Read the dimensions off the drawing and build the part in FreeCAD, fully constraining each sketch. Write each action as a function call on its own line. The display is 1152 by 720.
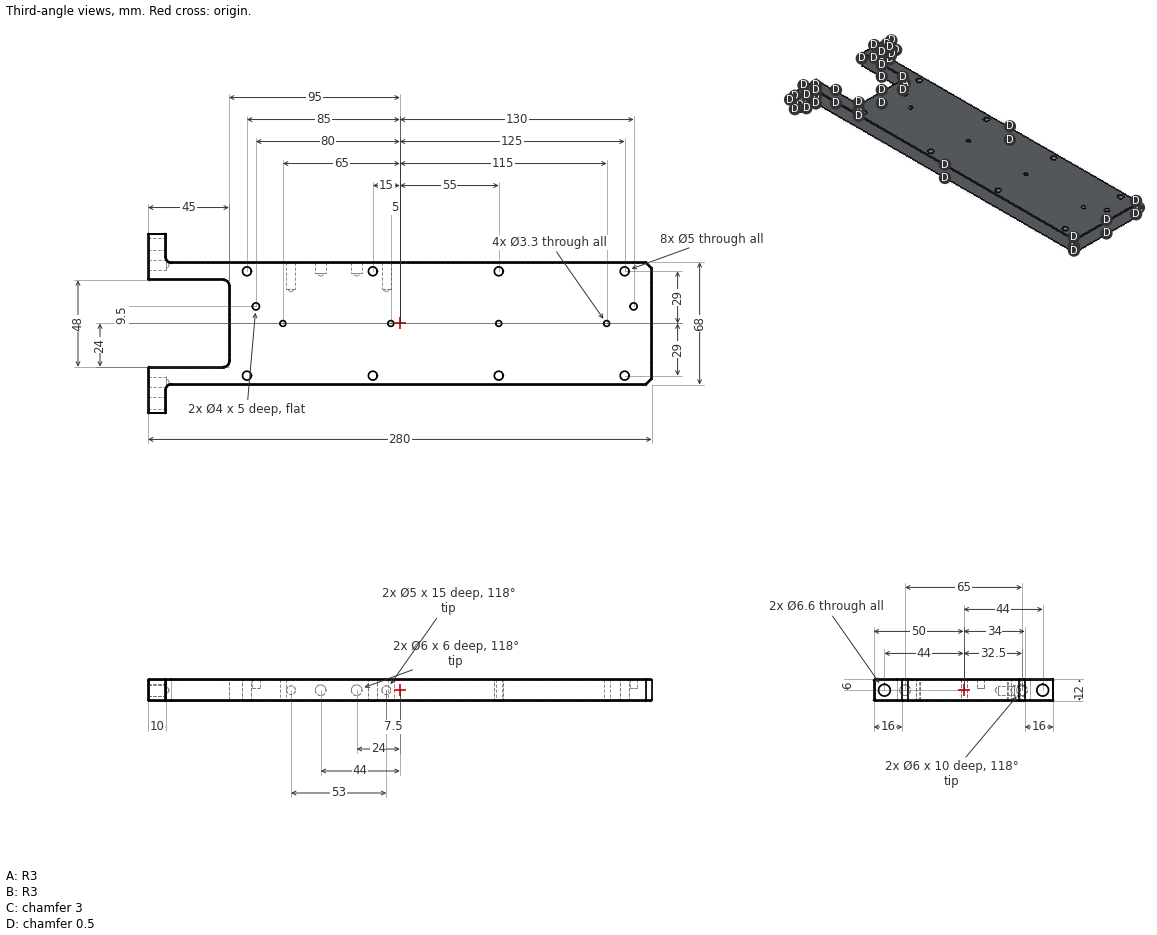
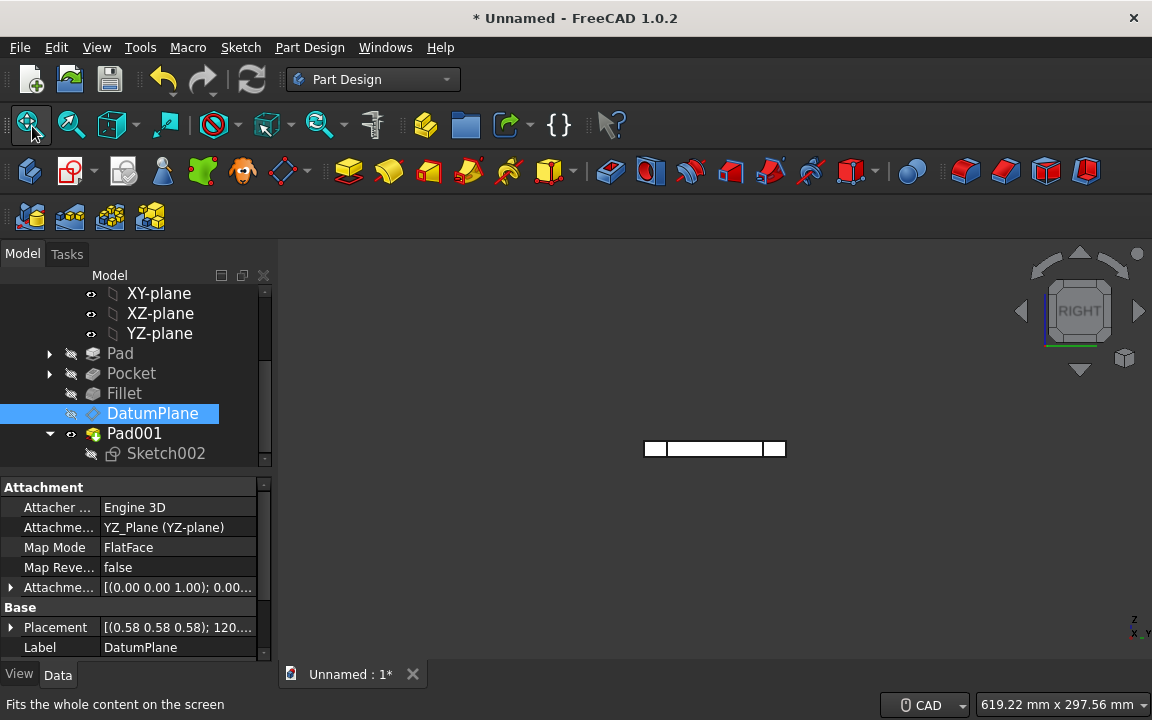
key(5)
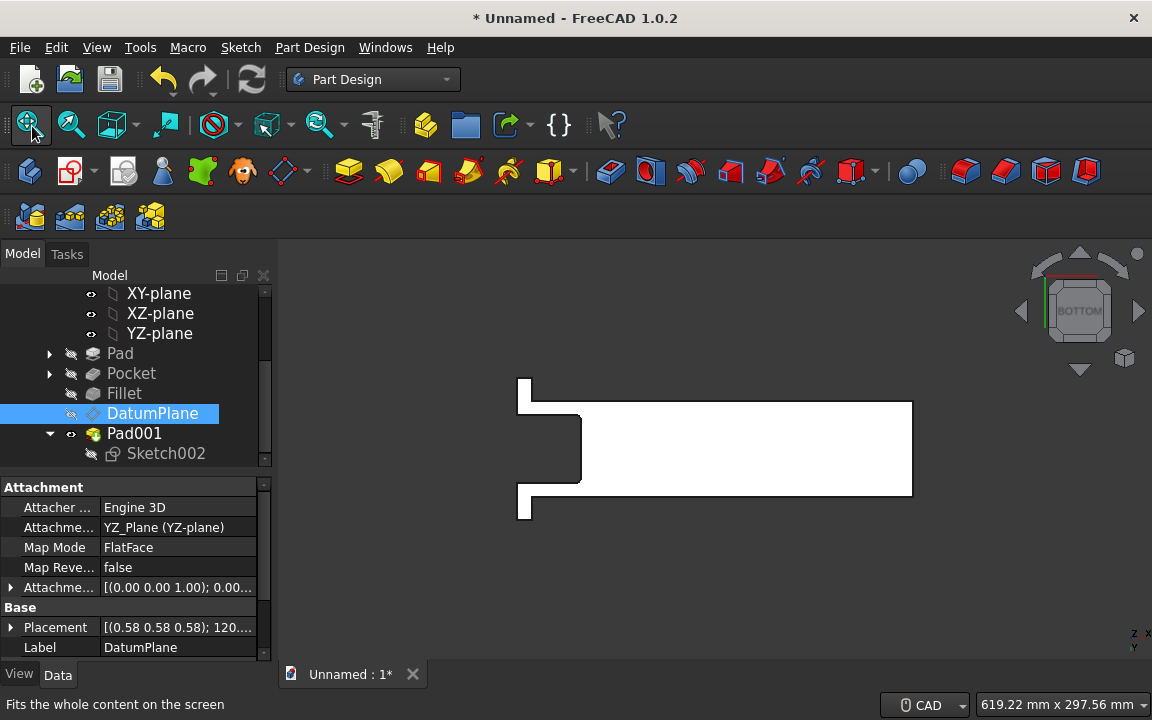
scroll(532, 400, up, 5)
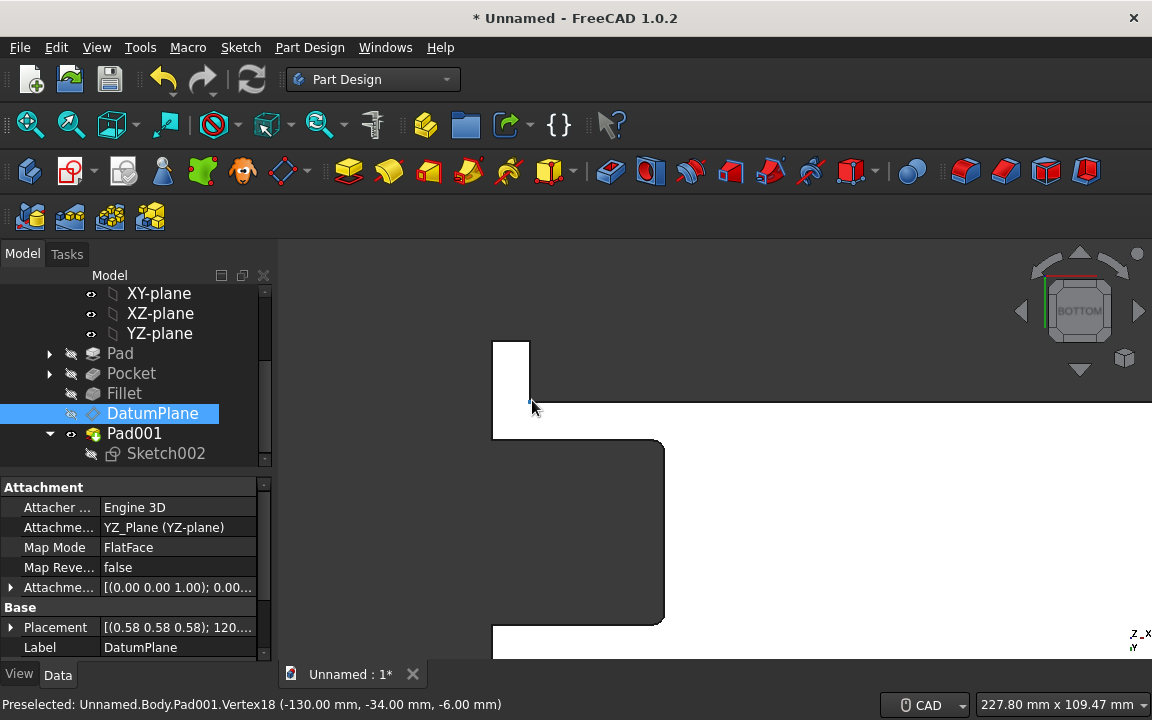
key(v)
key(f)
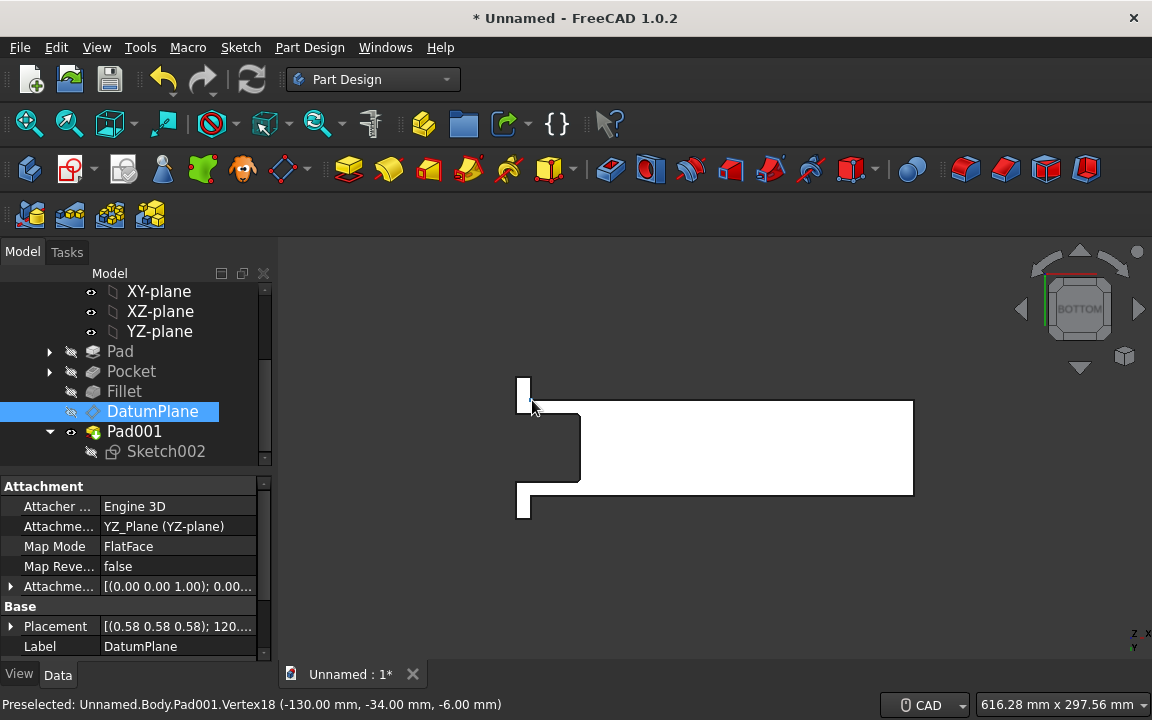
key(4)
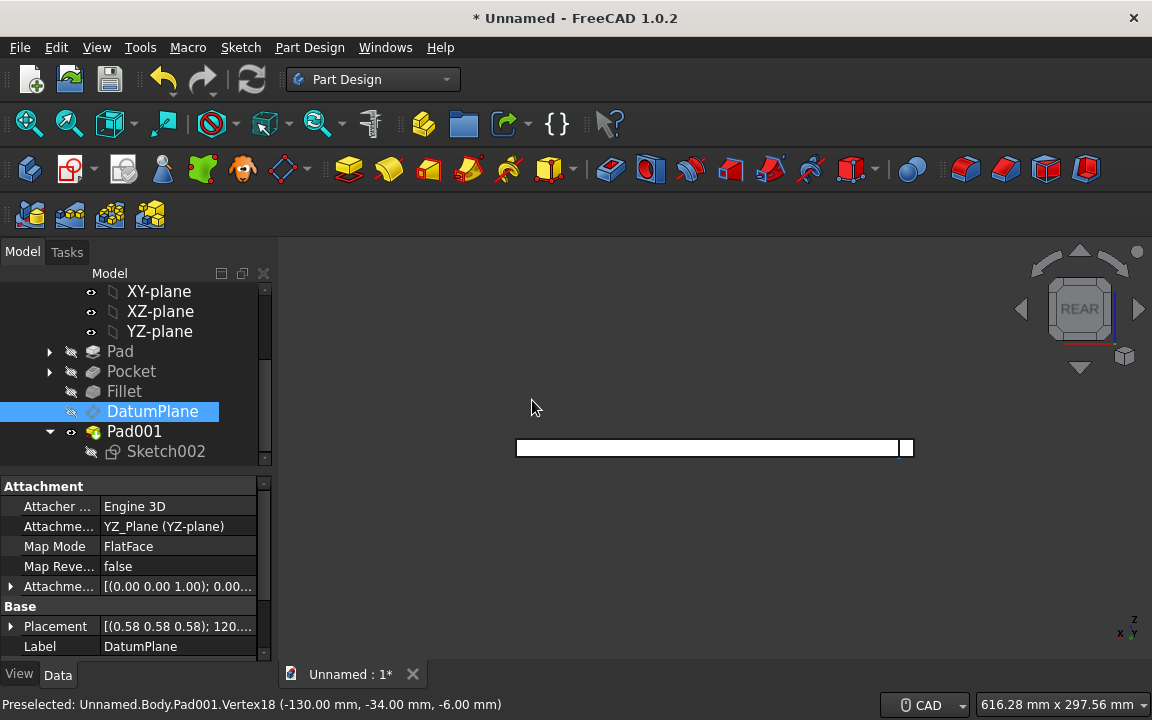
scroll(899, 447, up, 5)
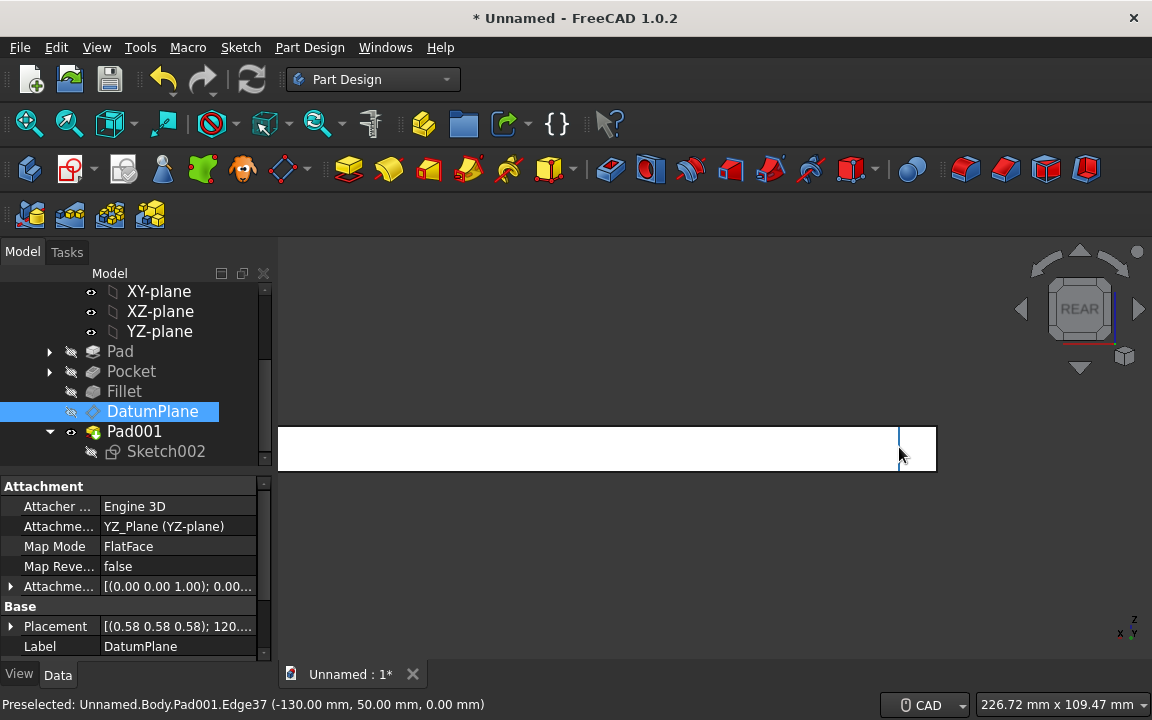
key(v)
key(f)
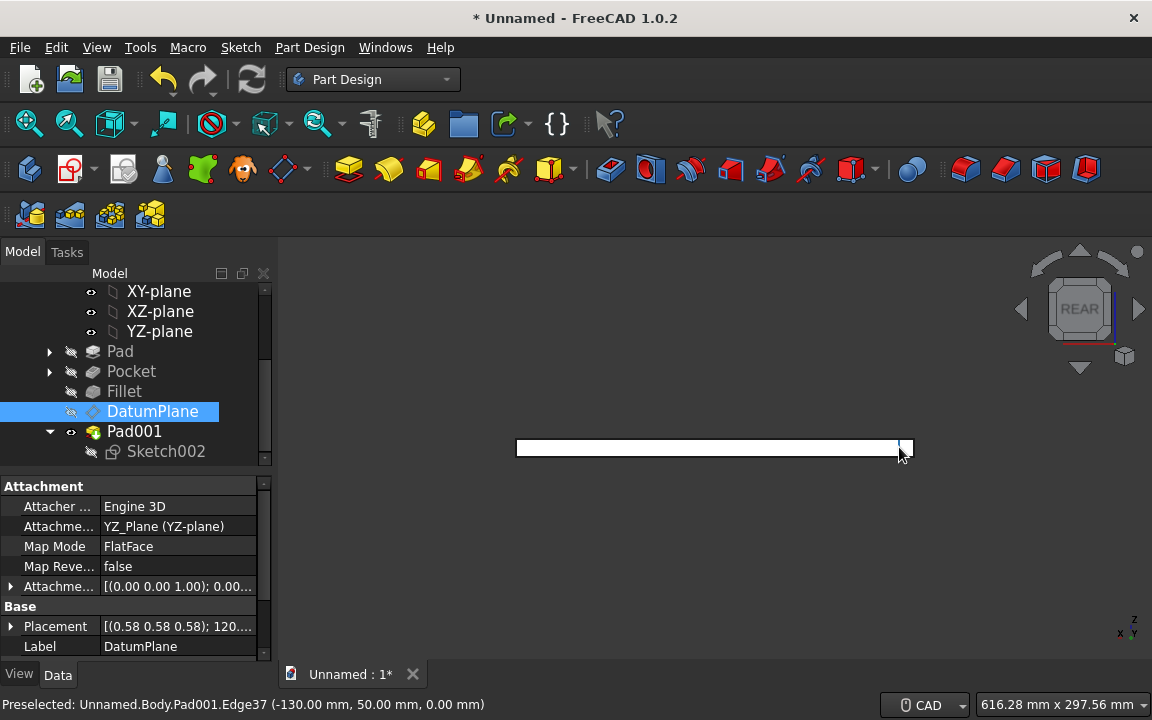
key(6)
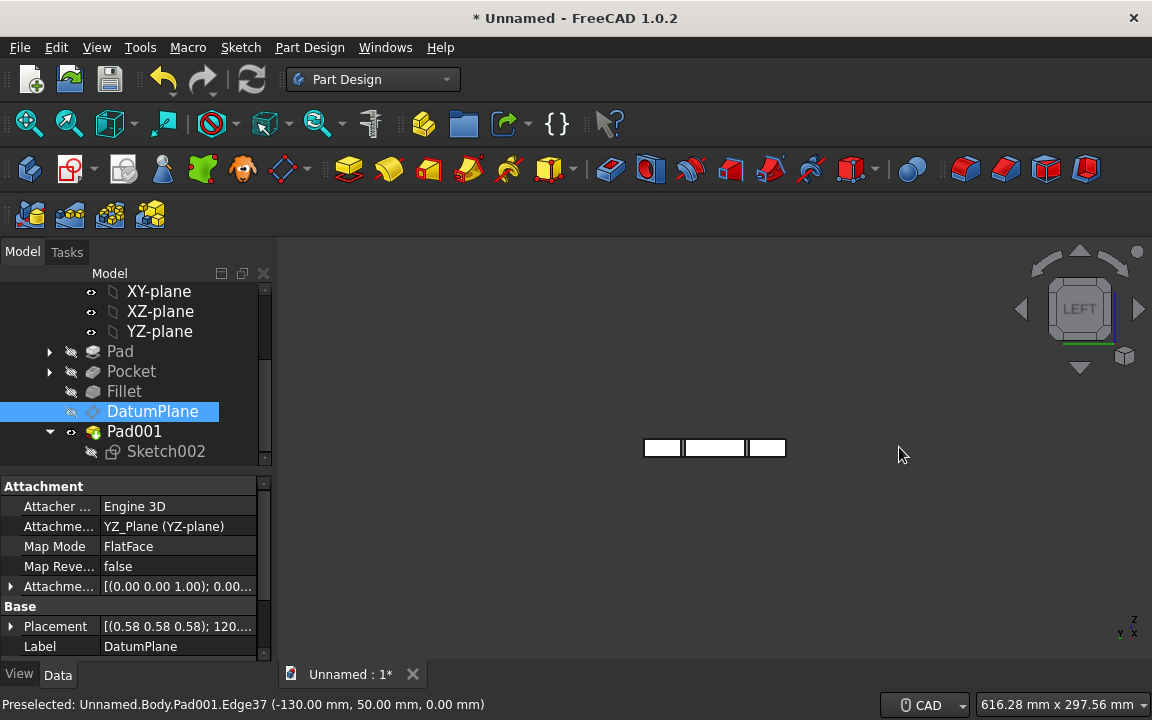
key(v)
key(f)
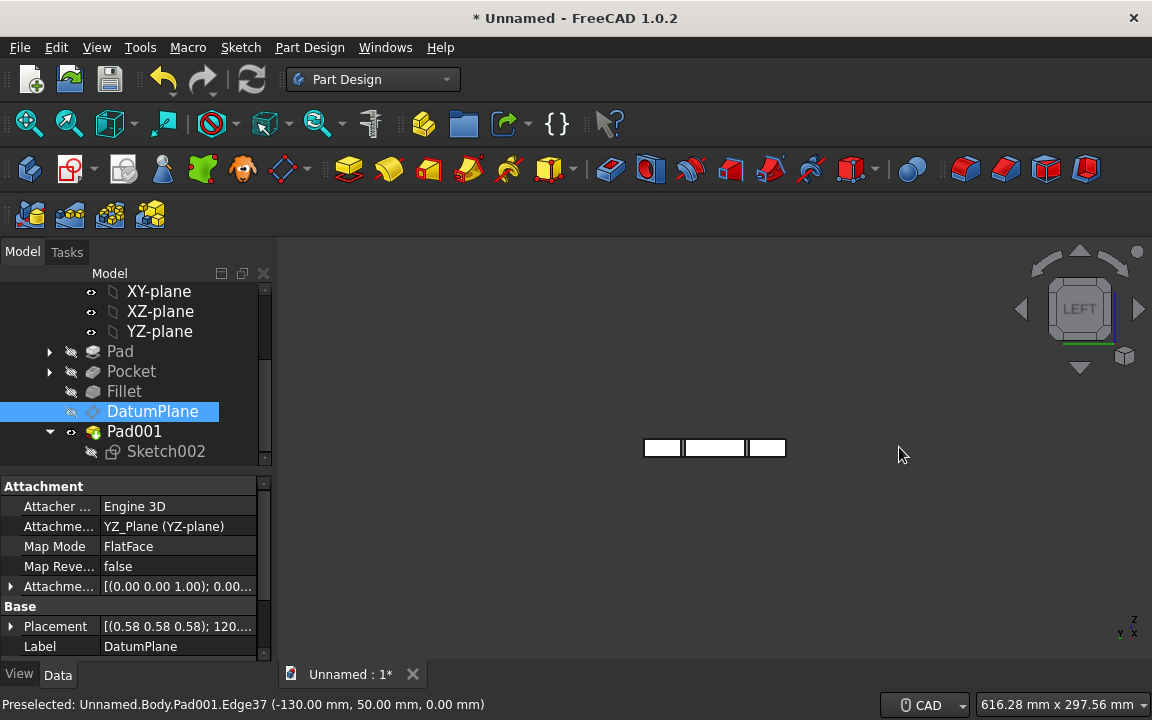
scroll(763, 447, up, 5)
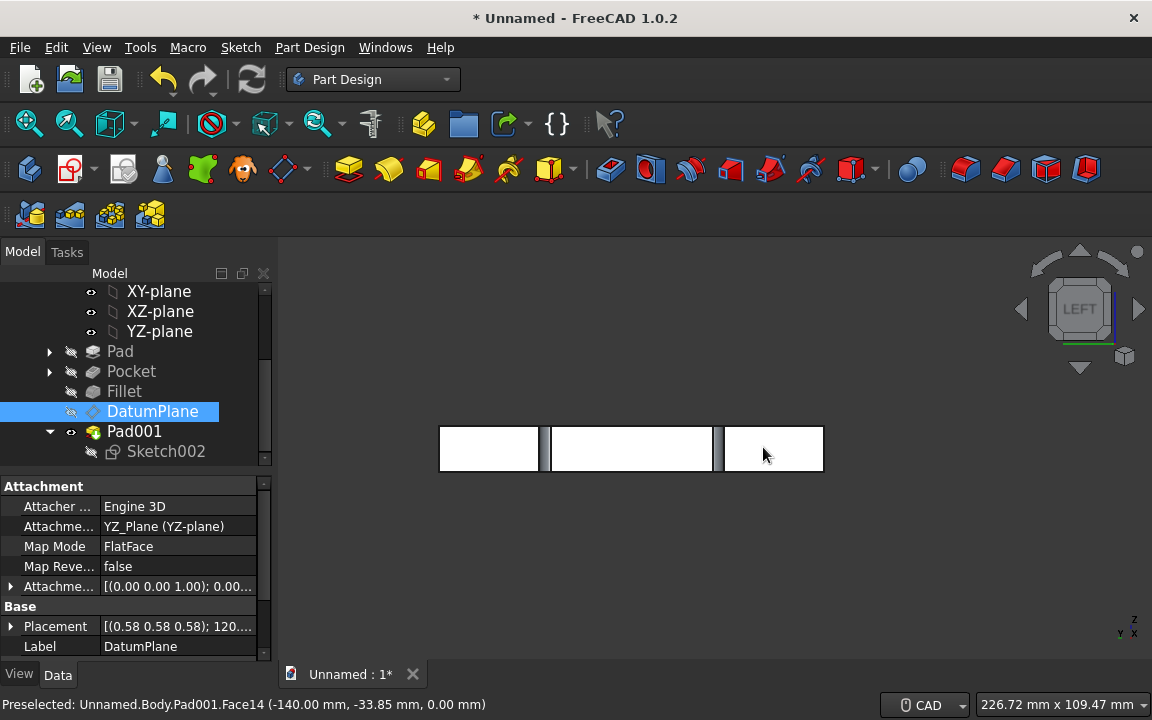
key(v)
key(f)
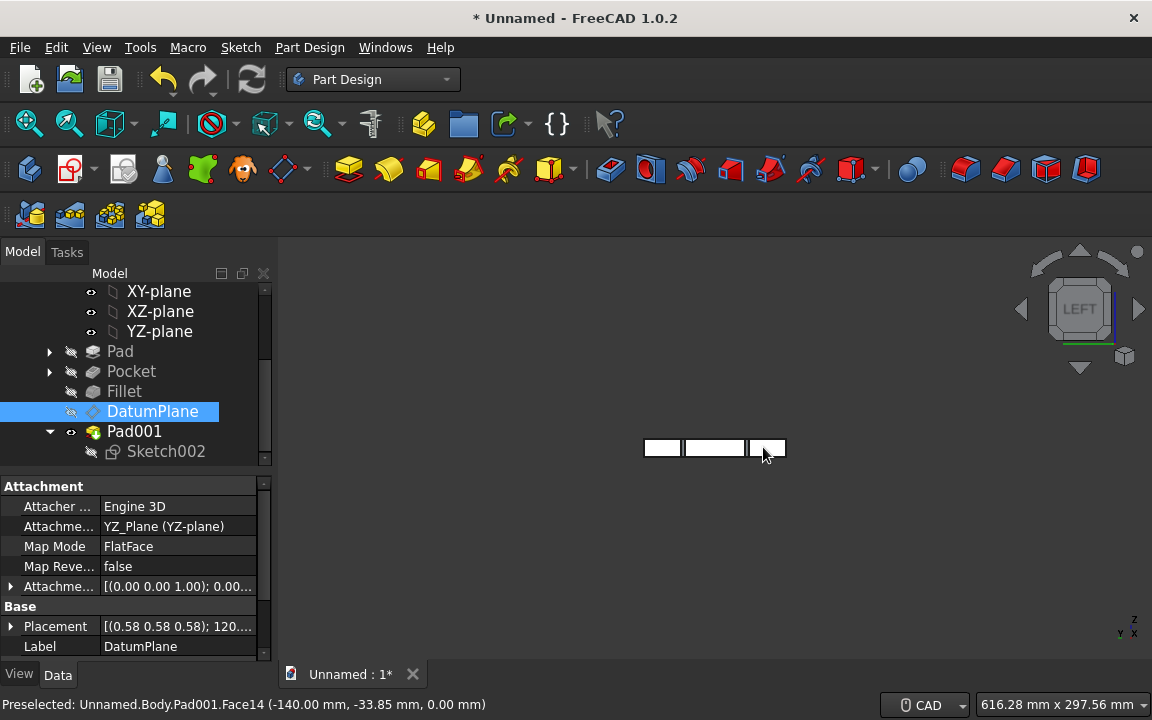
key(v)
key(3)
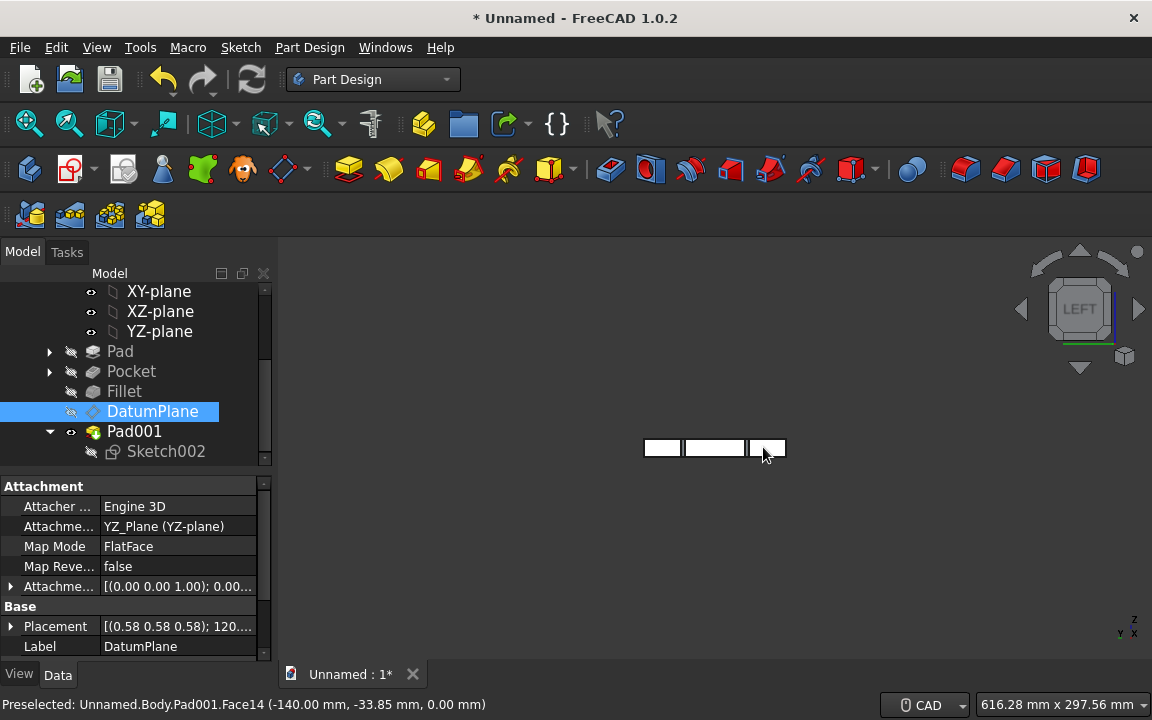
key(0)